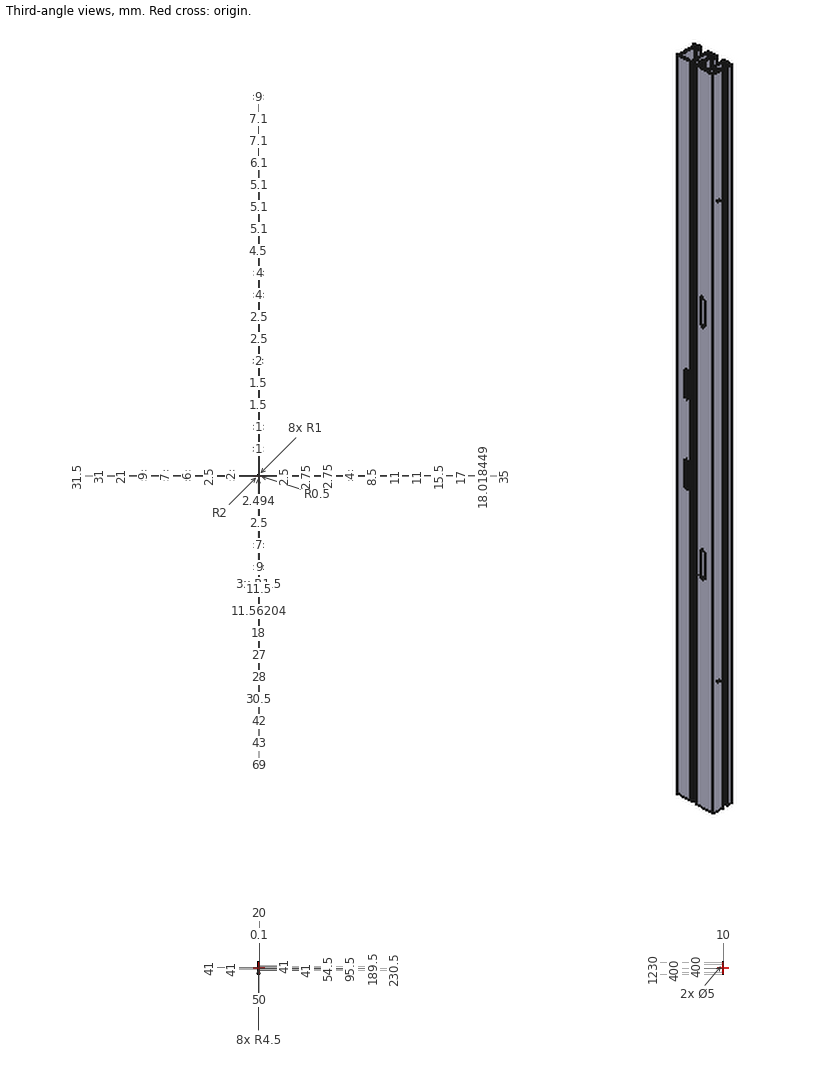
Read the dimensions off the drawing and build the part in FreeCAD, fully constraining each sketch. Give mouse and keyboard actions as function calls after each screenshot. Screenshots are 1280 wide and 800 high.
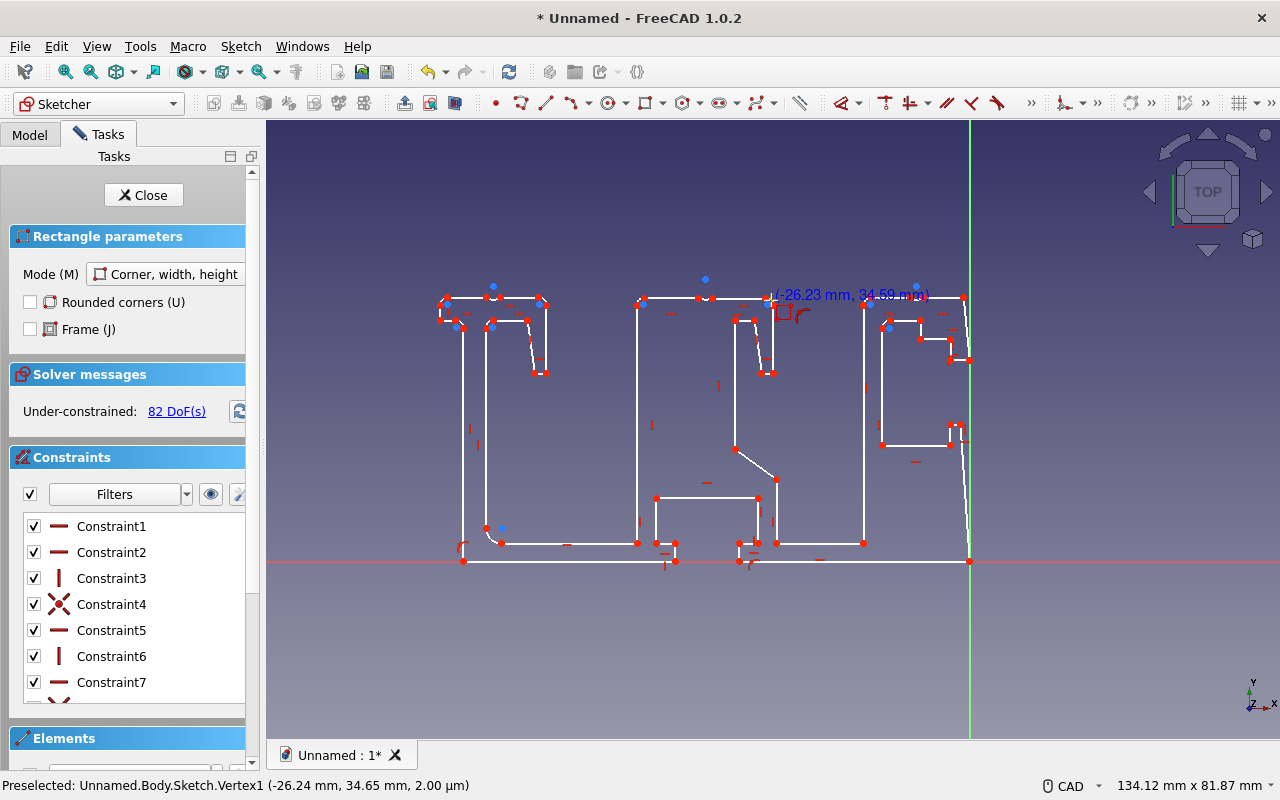
click(883, 460)
move(951, 543)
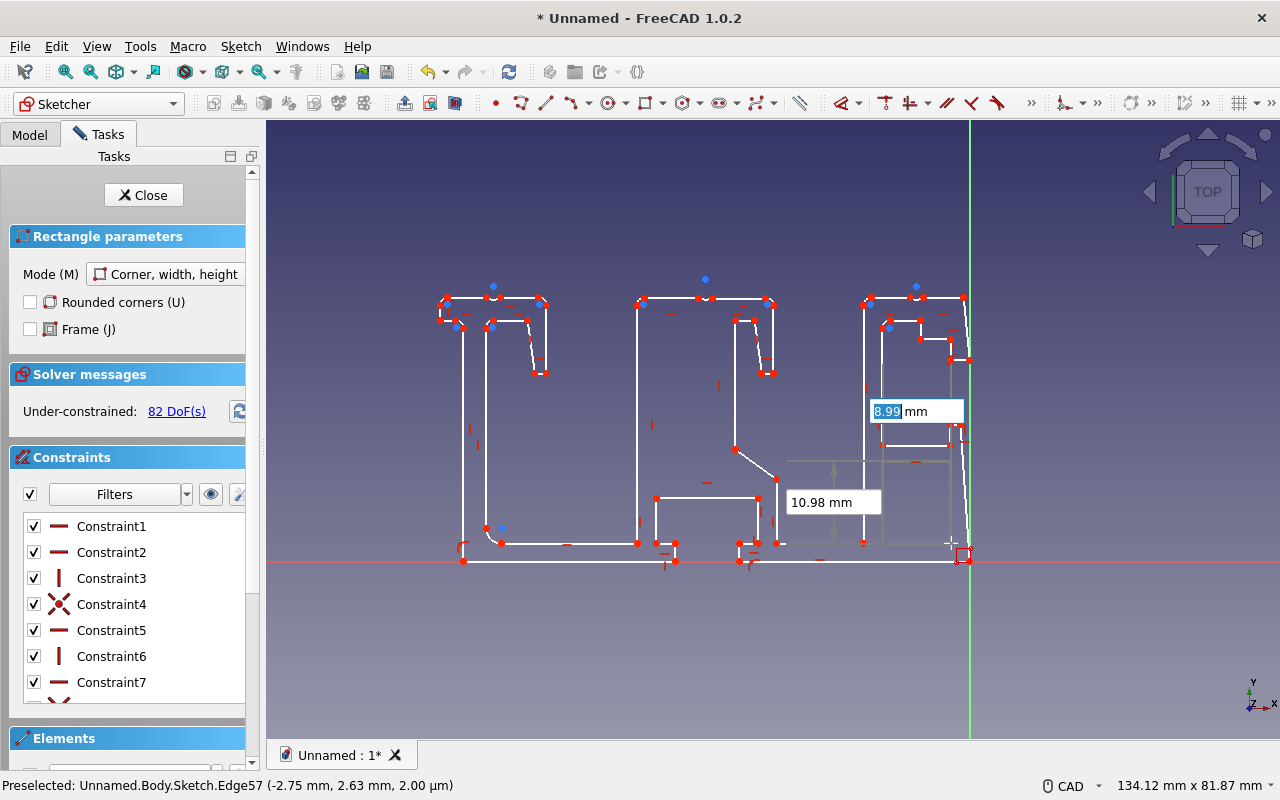
text(9)
key(Tab)
text(11)
key(Return)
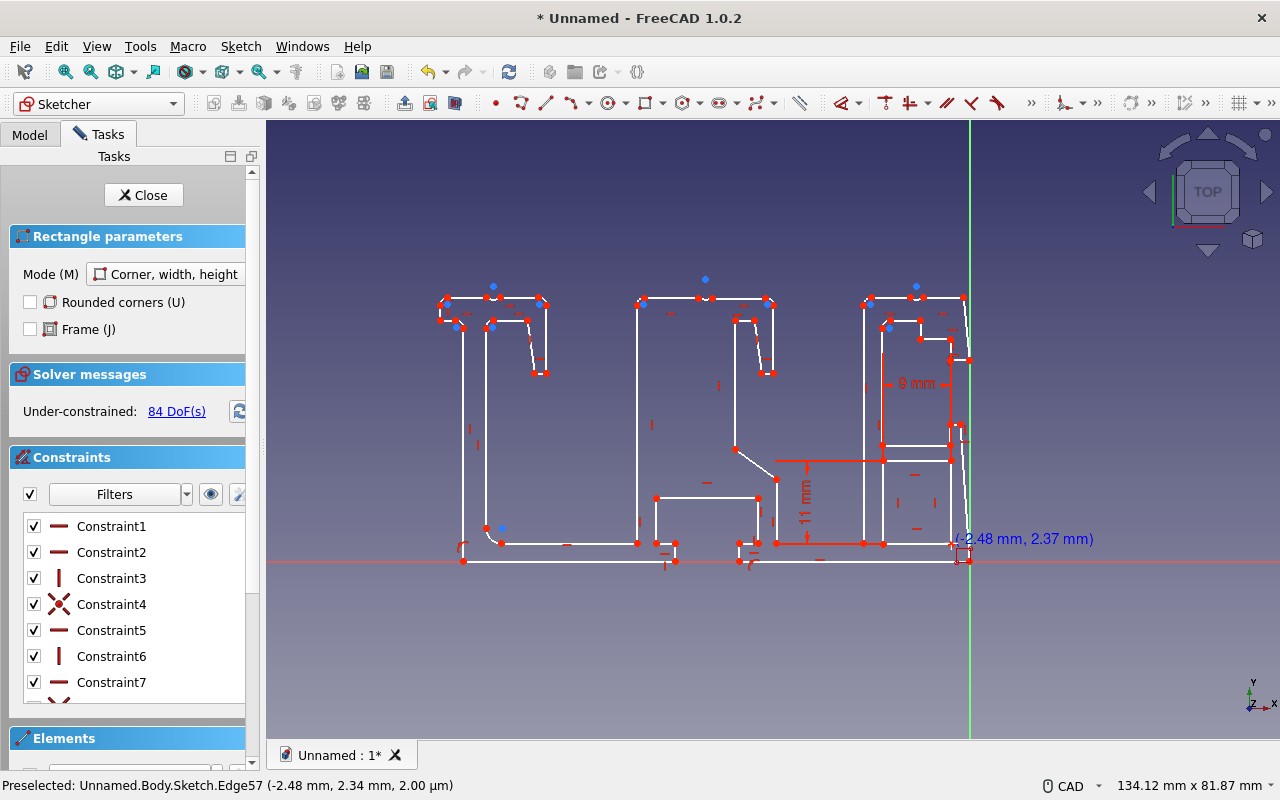
click(521, 104)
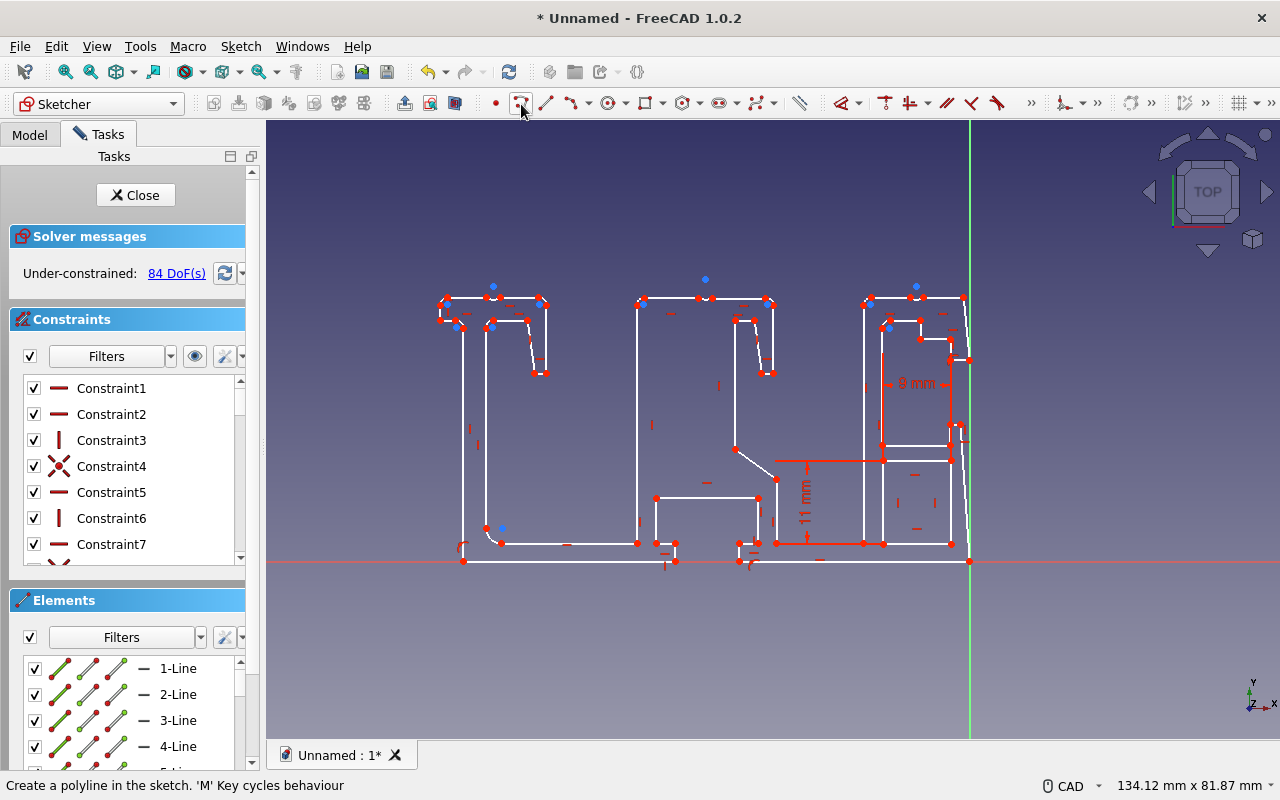
click(740, 479)
click(652, 479)
click(652, 320)
click(720, 320)
click(720, 456)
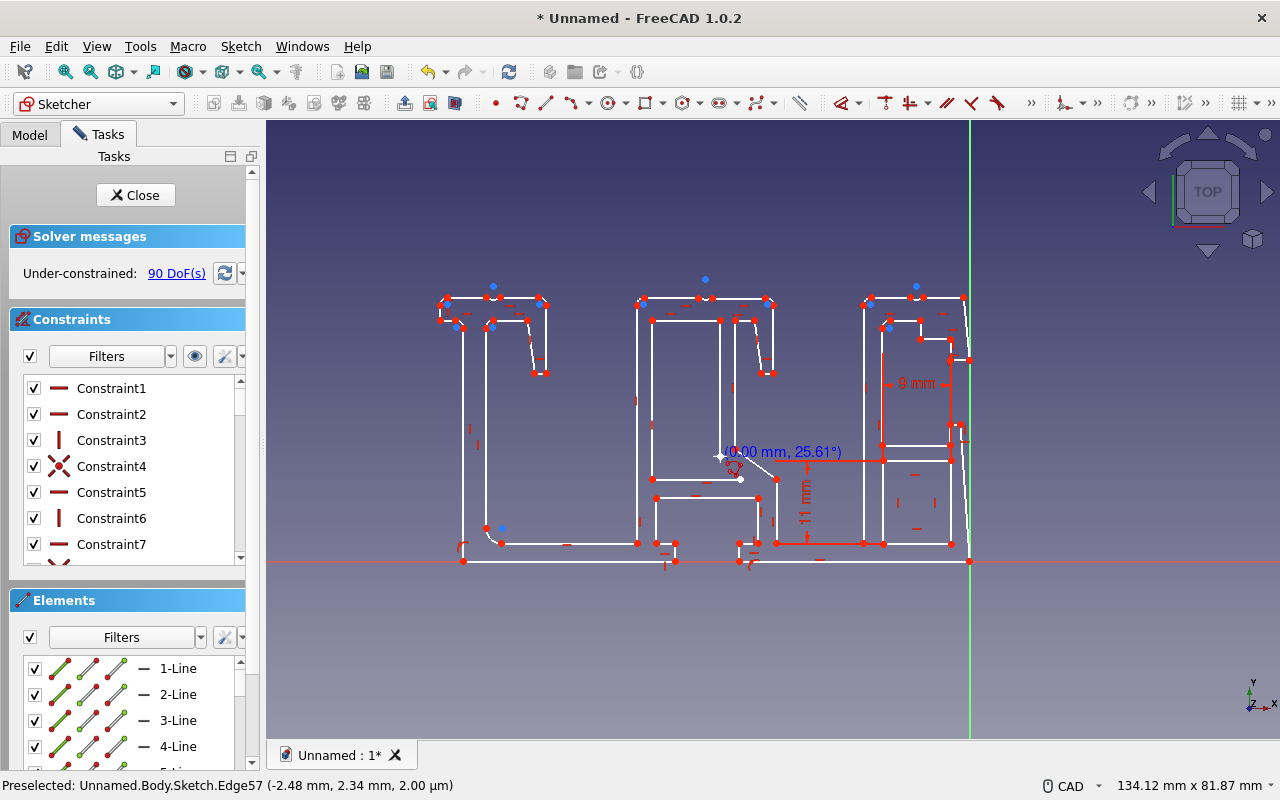
scroll(742, 472, up, 4)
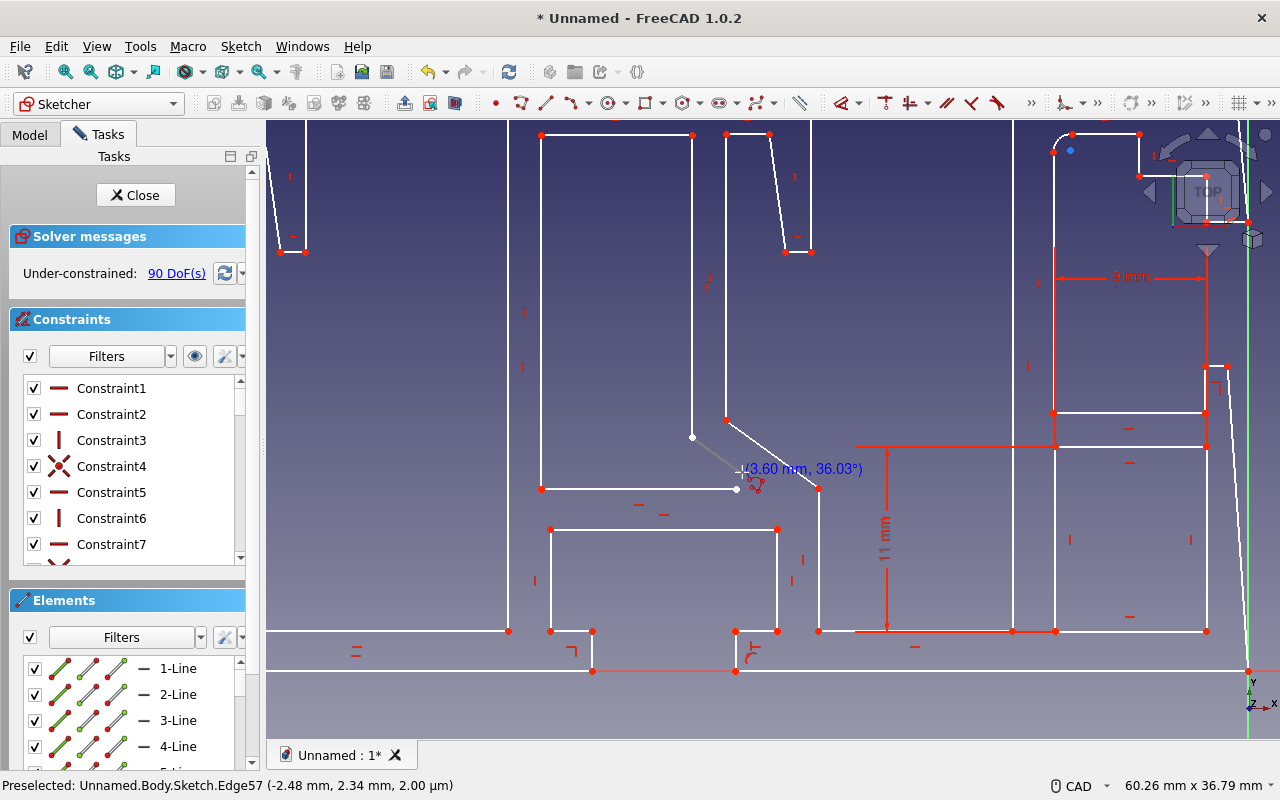
click(741, 471)
right_click(741, 471)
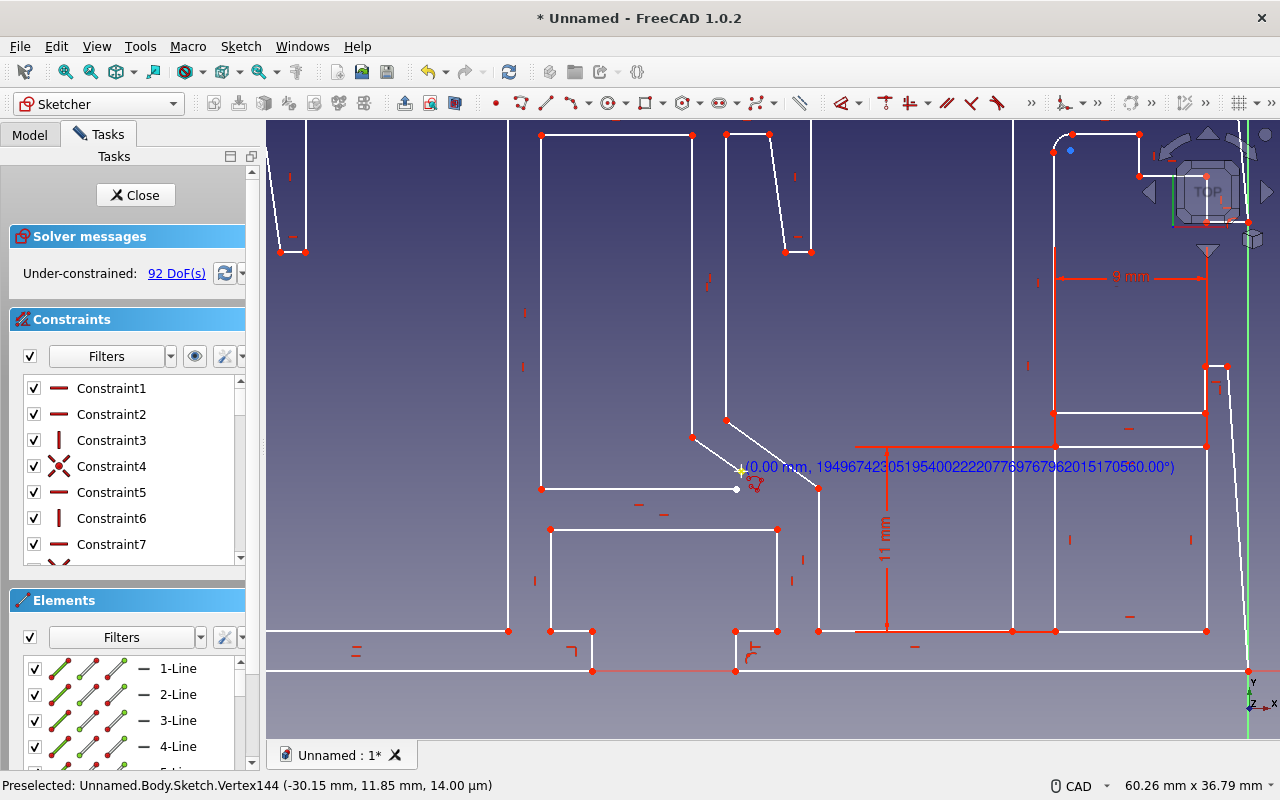
click(570, 104)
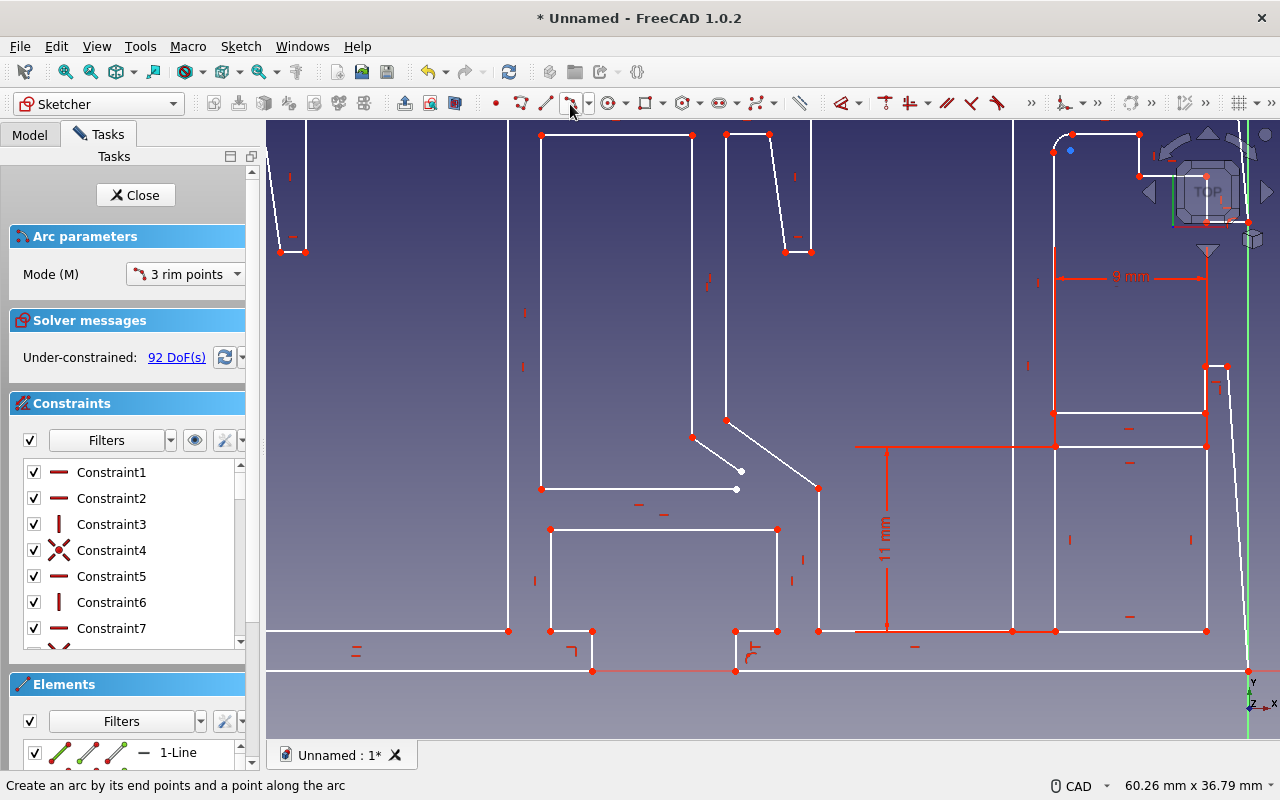
click(741, 472)
click(737, 489)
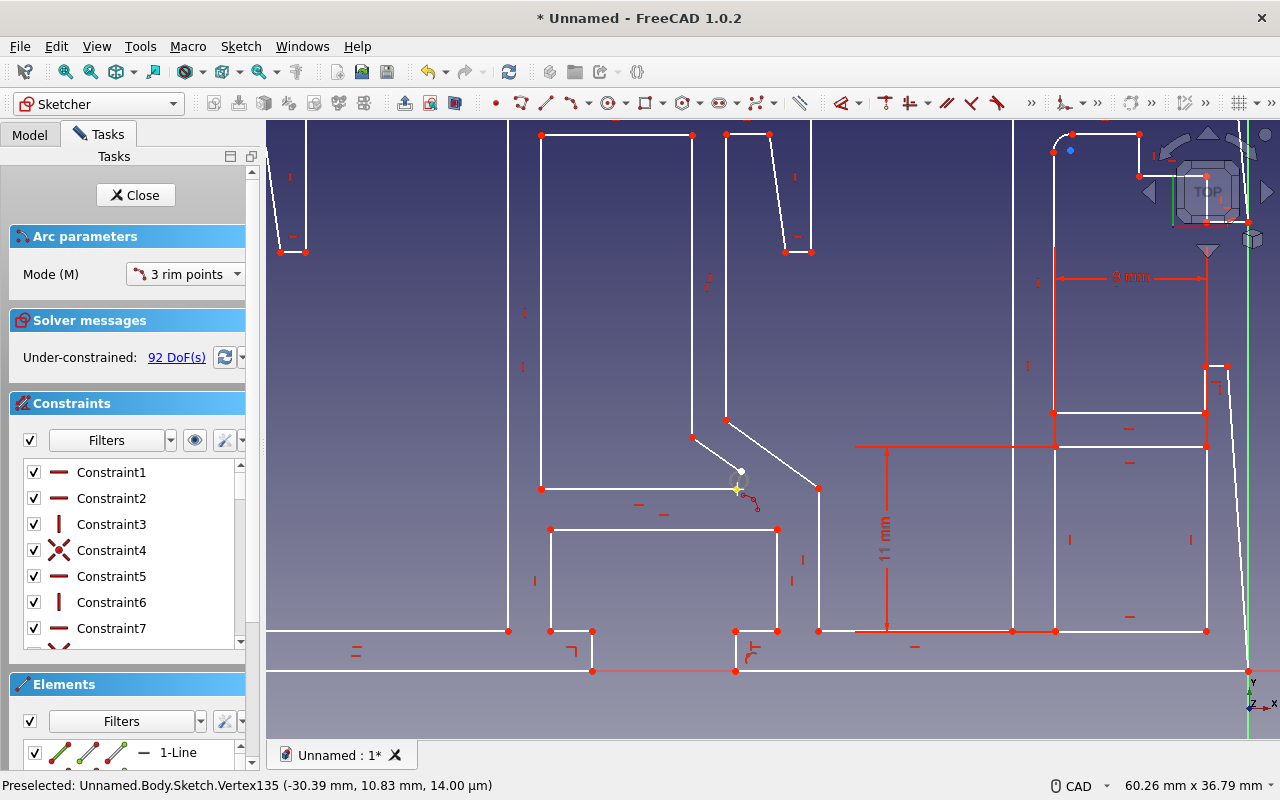
scroll(744, 480, up, 6)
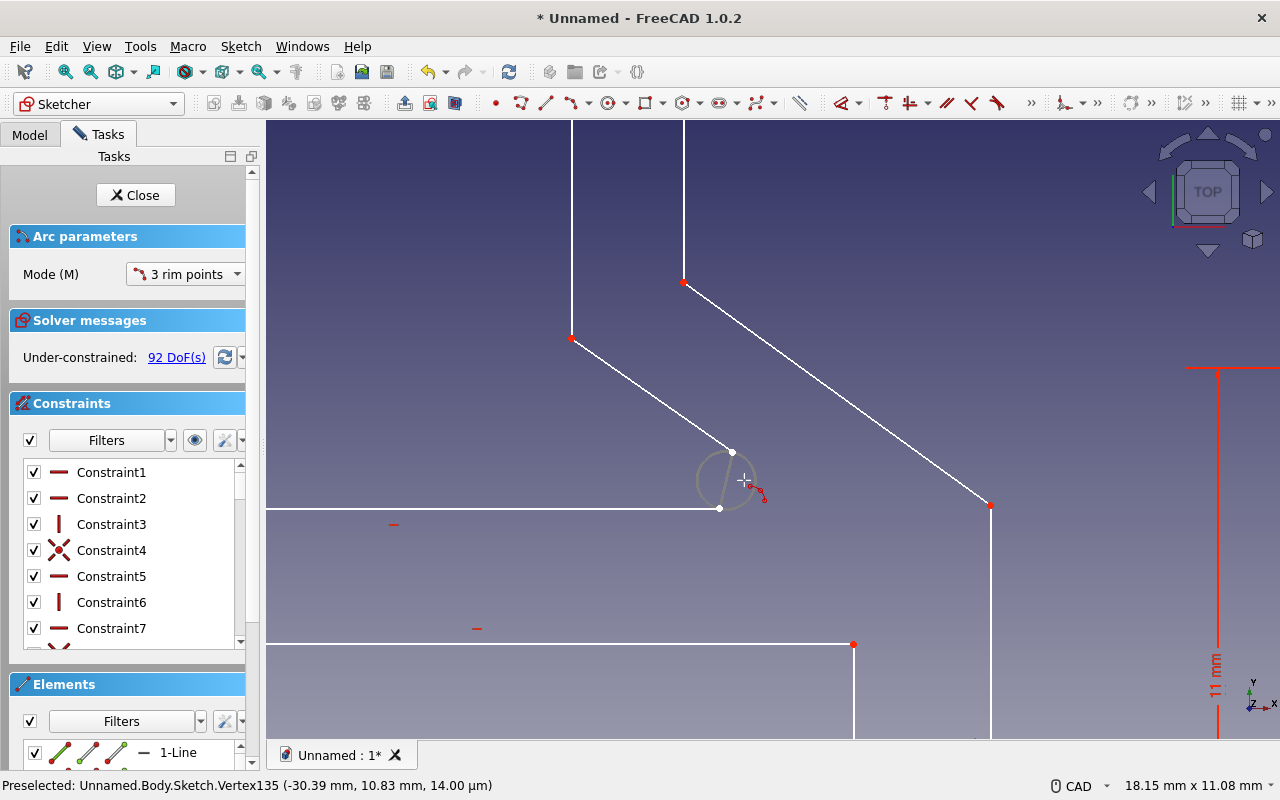
click(743, 480)
key(Escape)